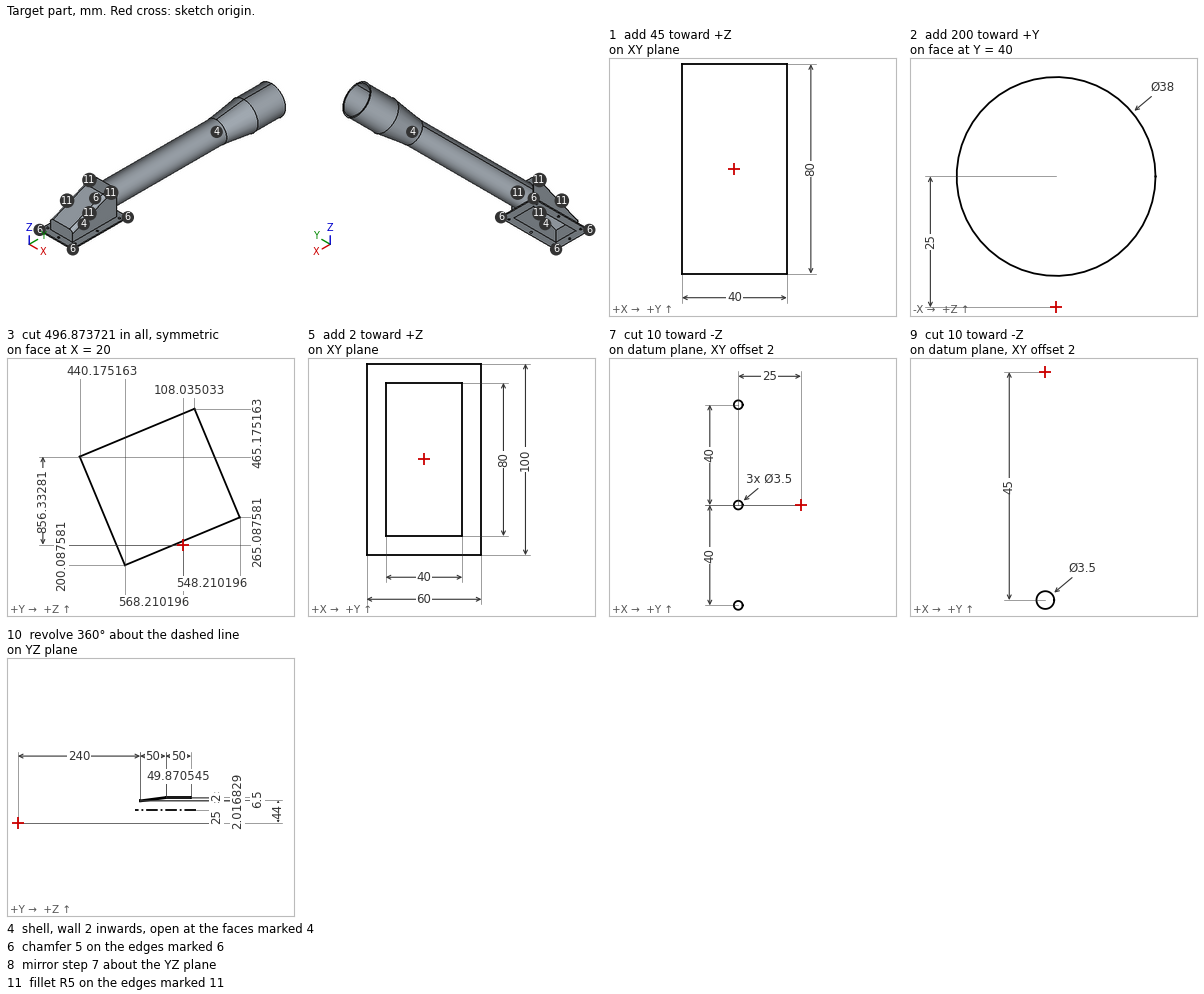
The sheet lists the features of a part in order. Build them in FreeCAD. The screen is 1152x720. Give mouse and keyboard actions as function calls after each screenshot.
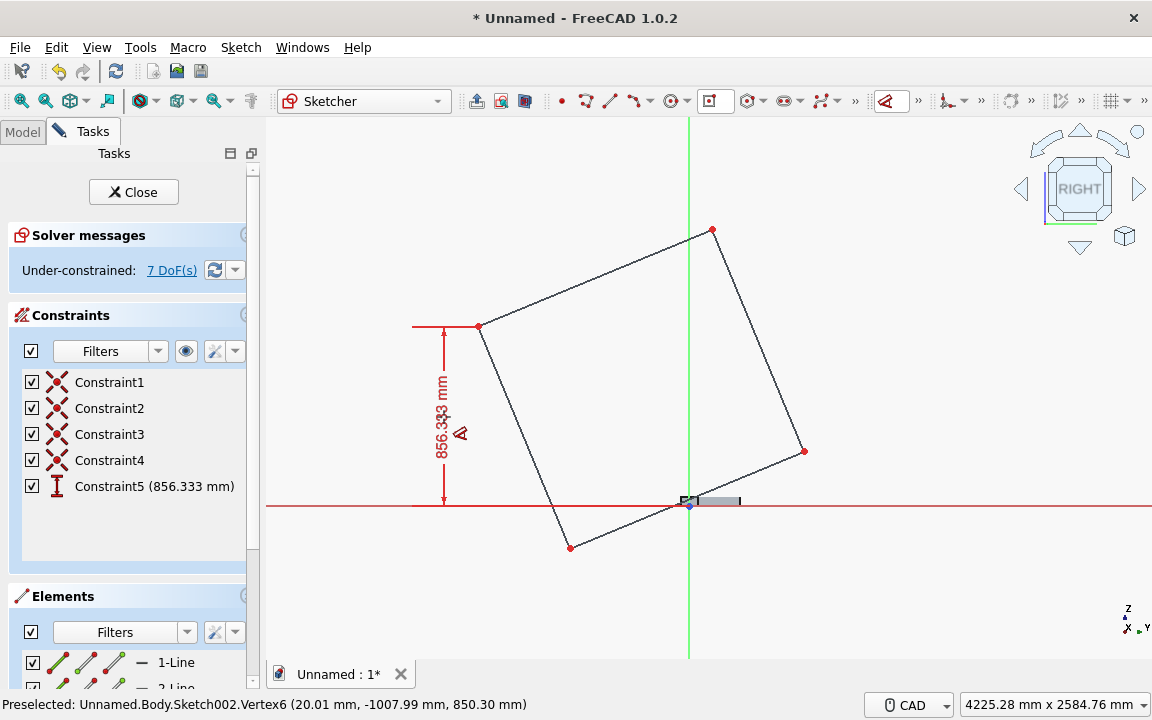
click(570, 549)
click(630, 583)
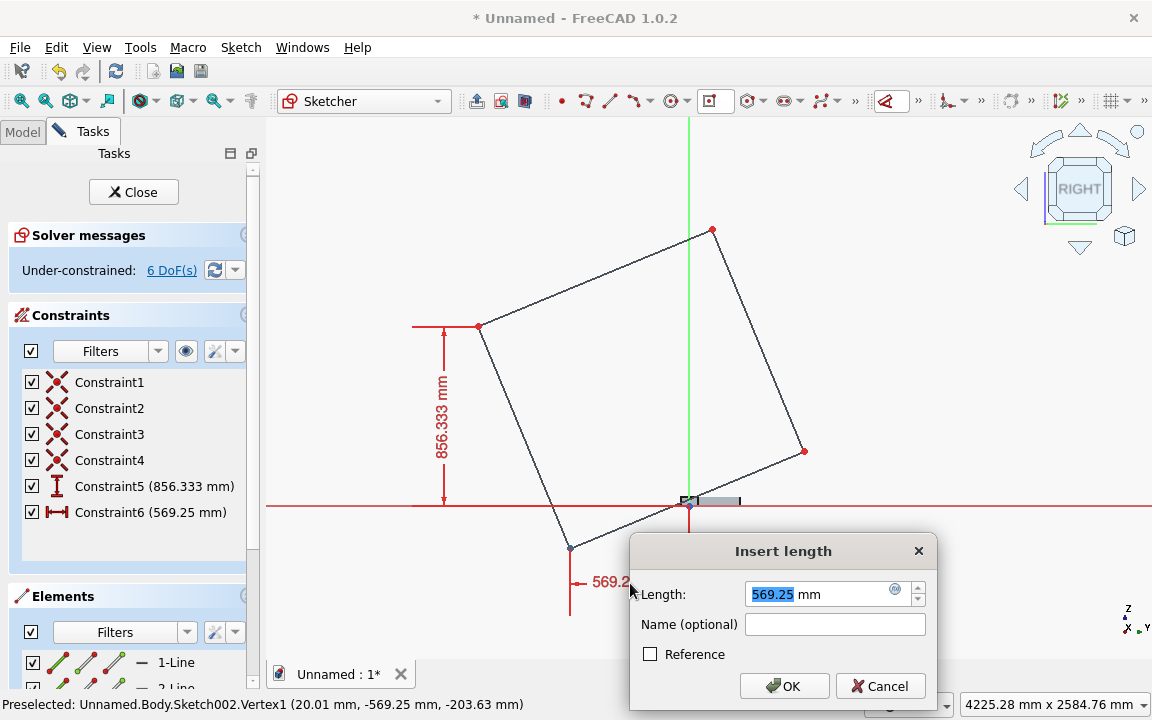
text(568.210196)
key(Return)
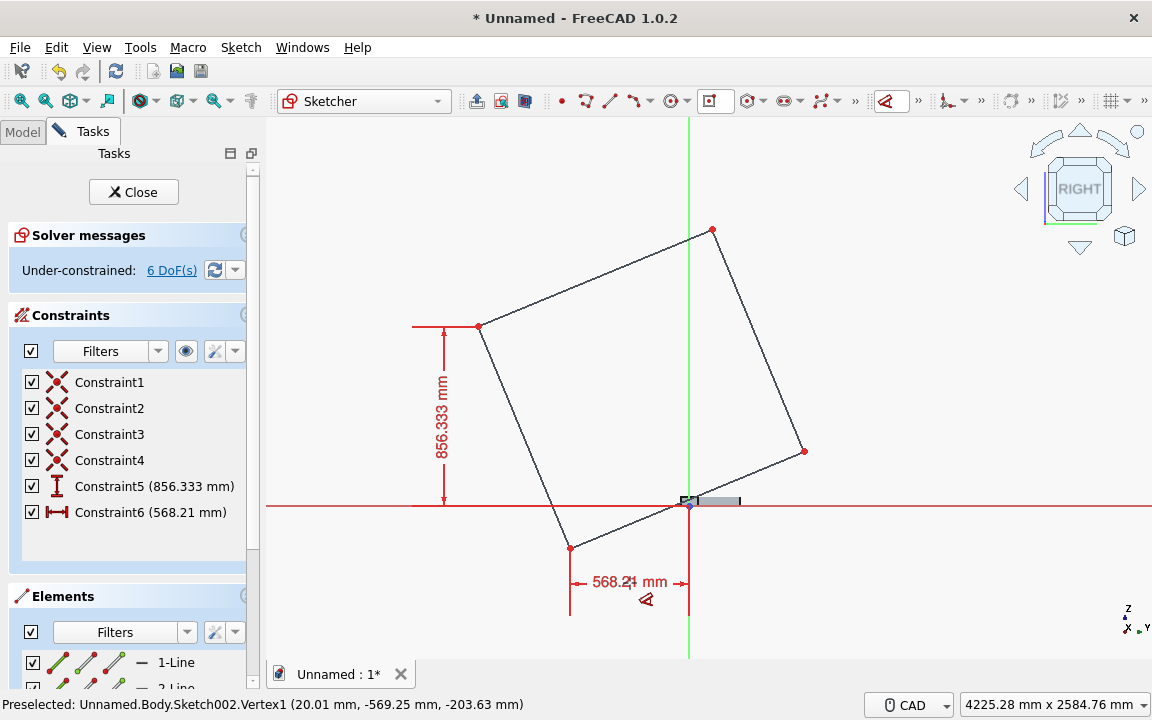
click(570, 549)
click(536, 528)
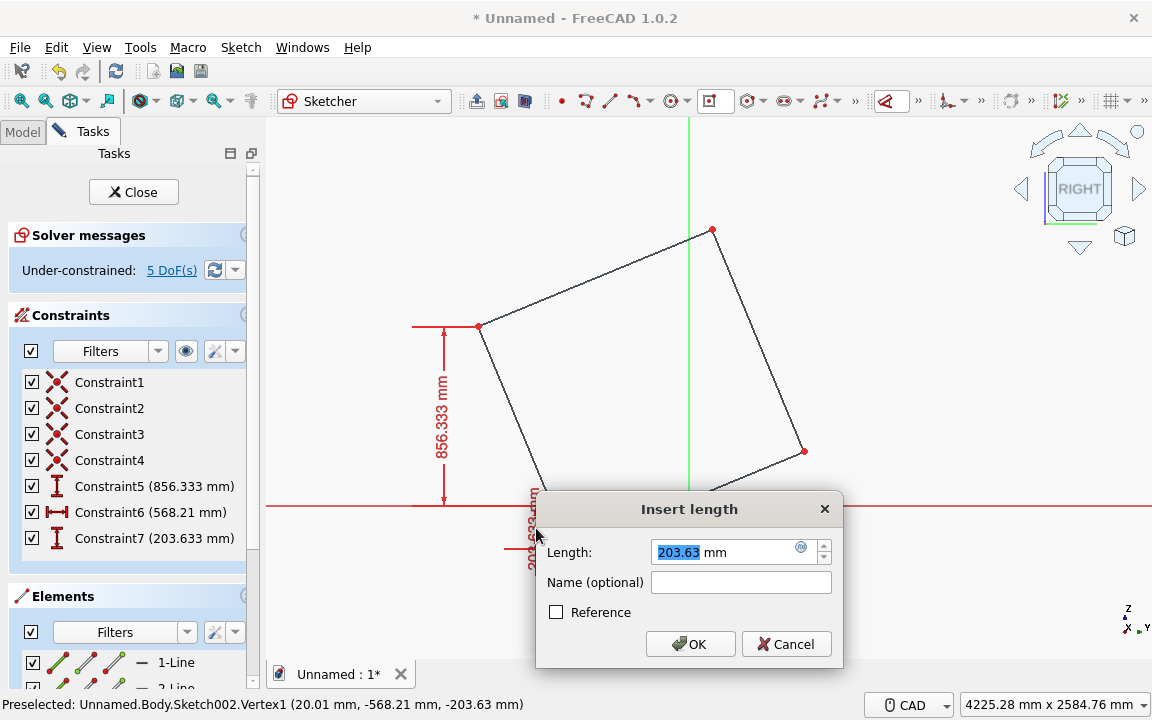
text(200.087581)
key(Return)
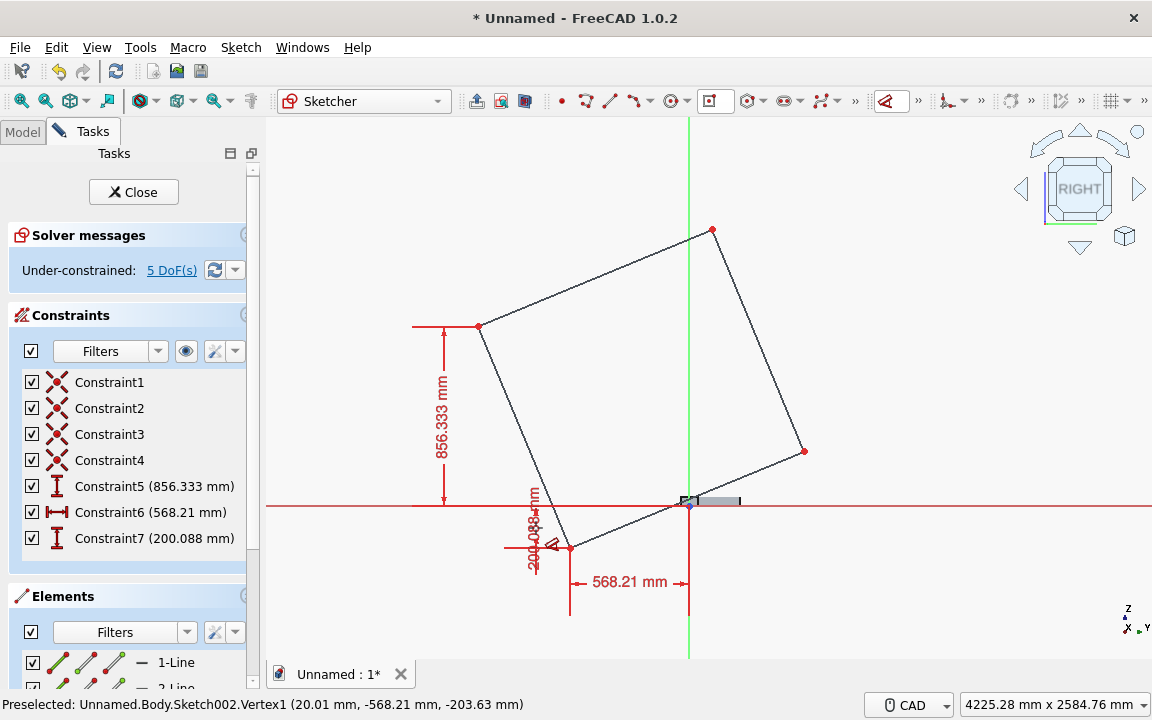
click(804, 452)
click(747, 540)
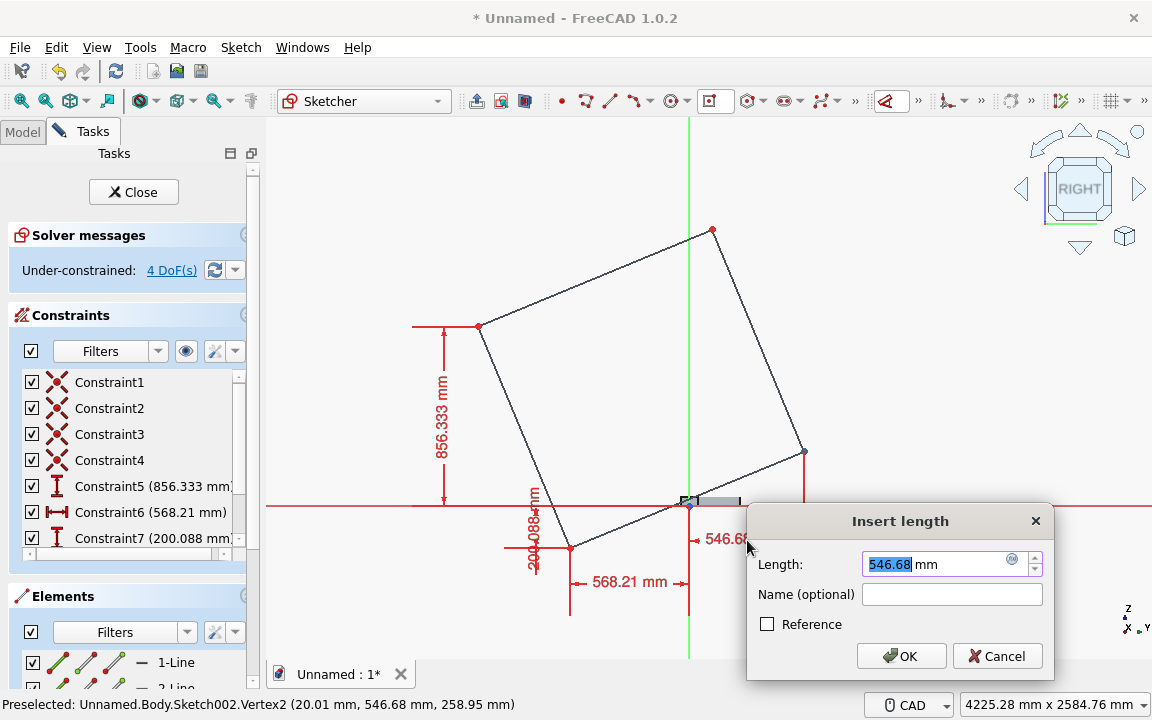
text(548.210196)
key(Return)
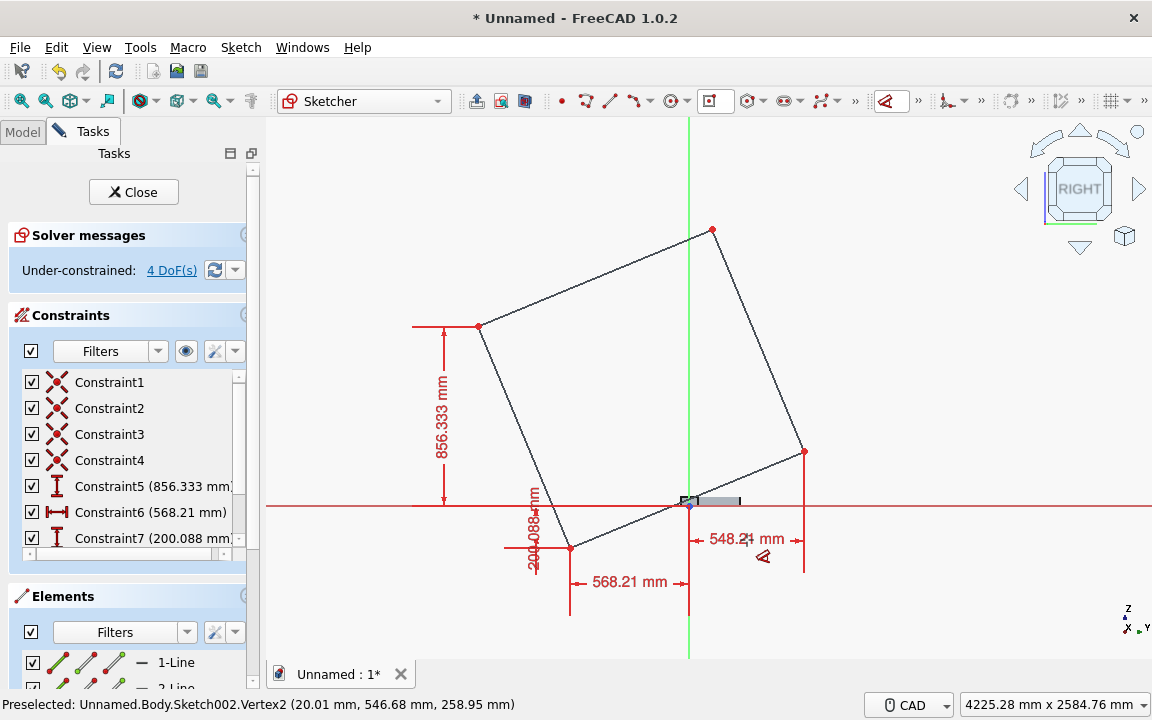
click(804, 452)
click(838, 479)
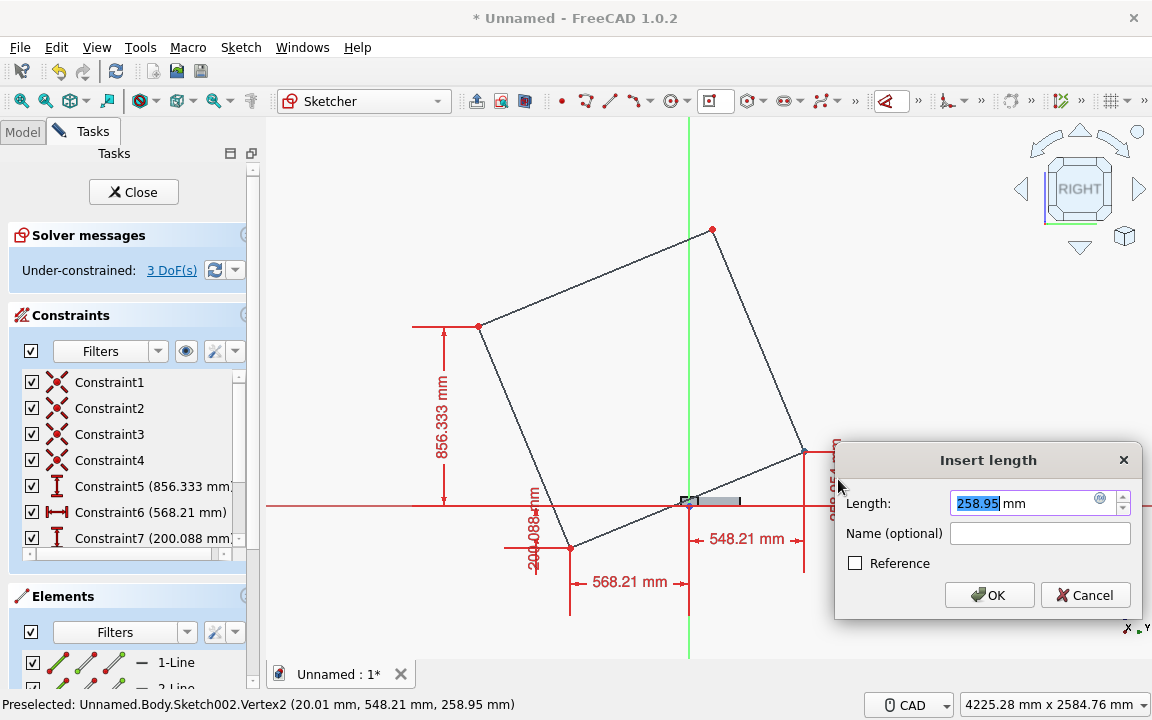
text(265.087581)
key(Return)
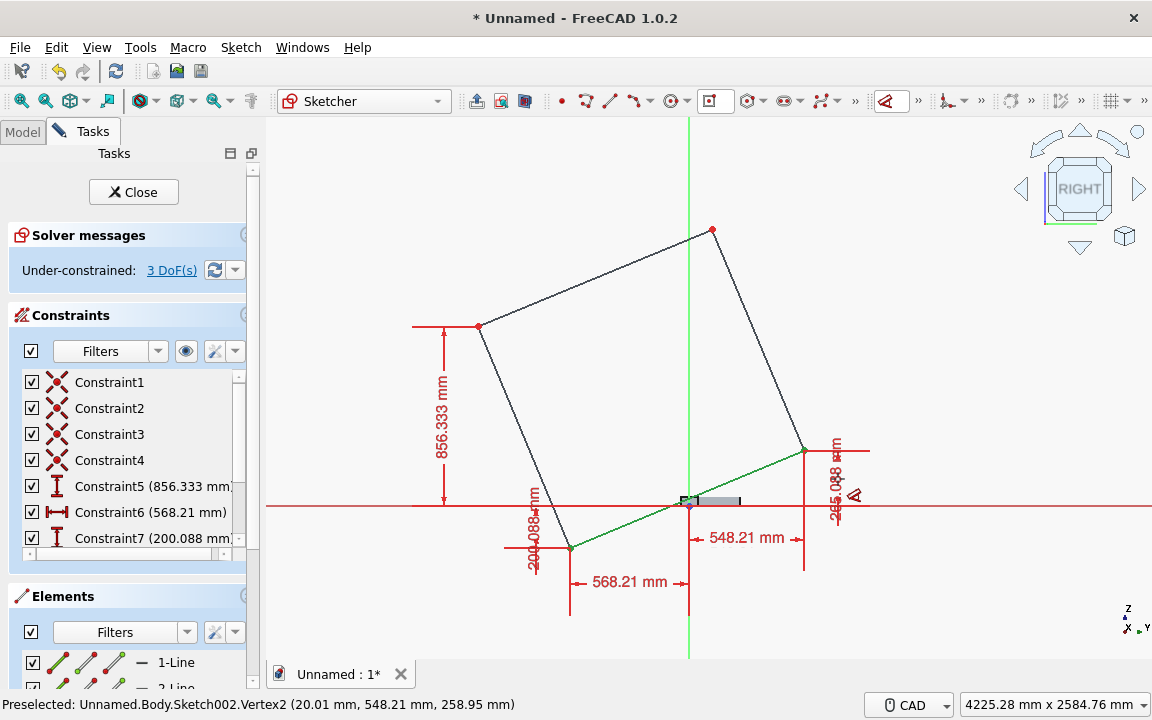
scroll(712, 230, up, 3)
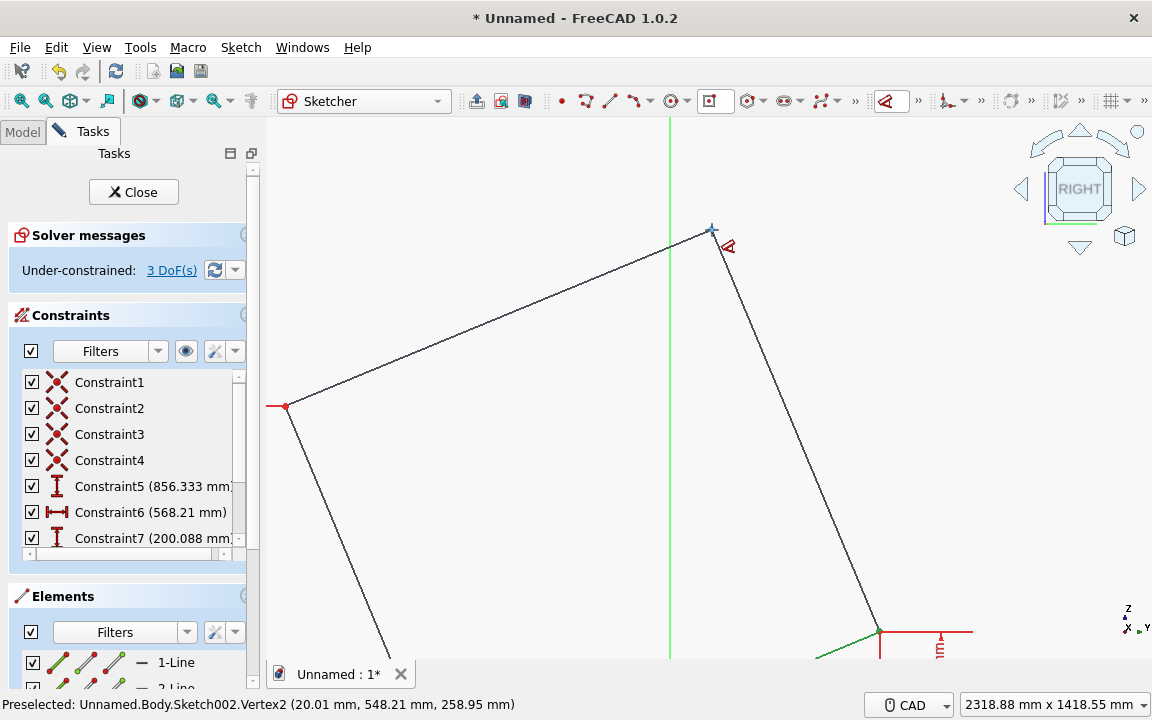
click(712, 230)
click(691, 196)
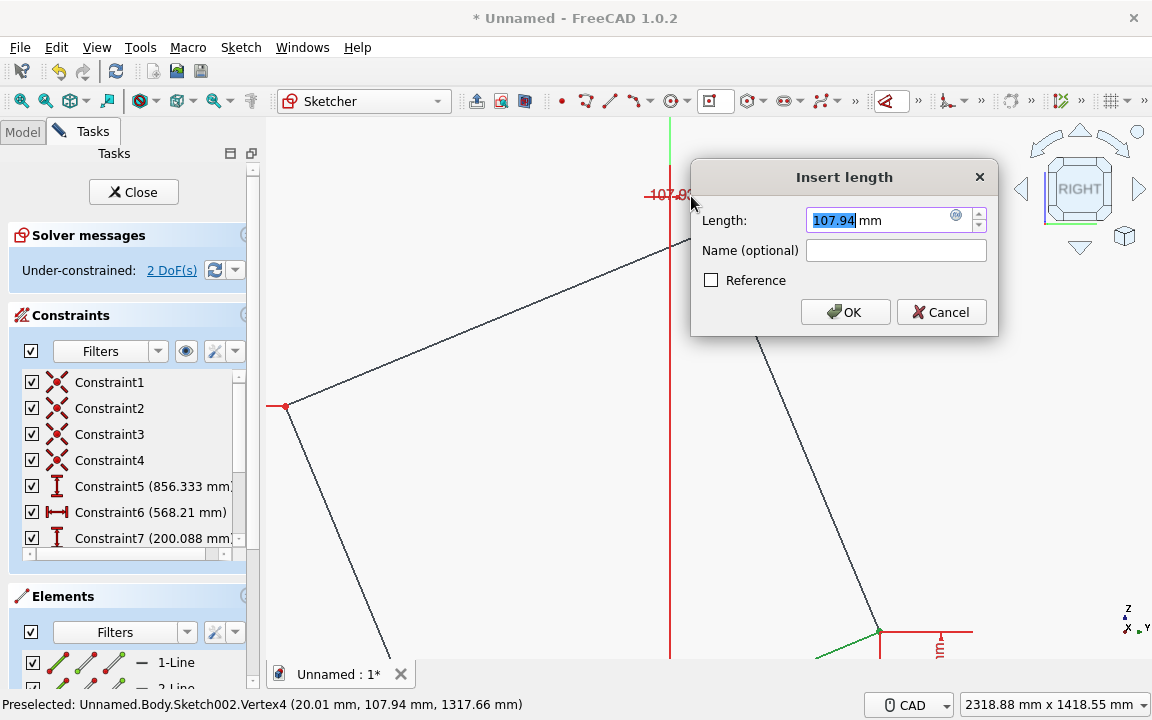
text(108.035033)
key(Return)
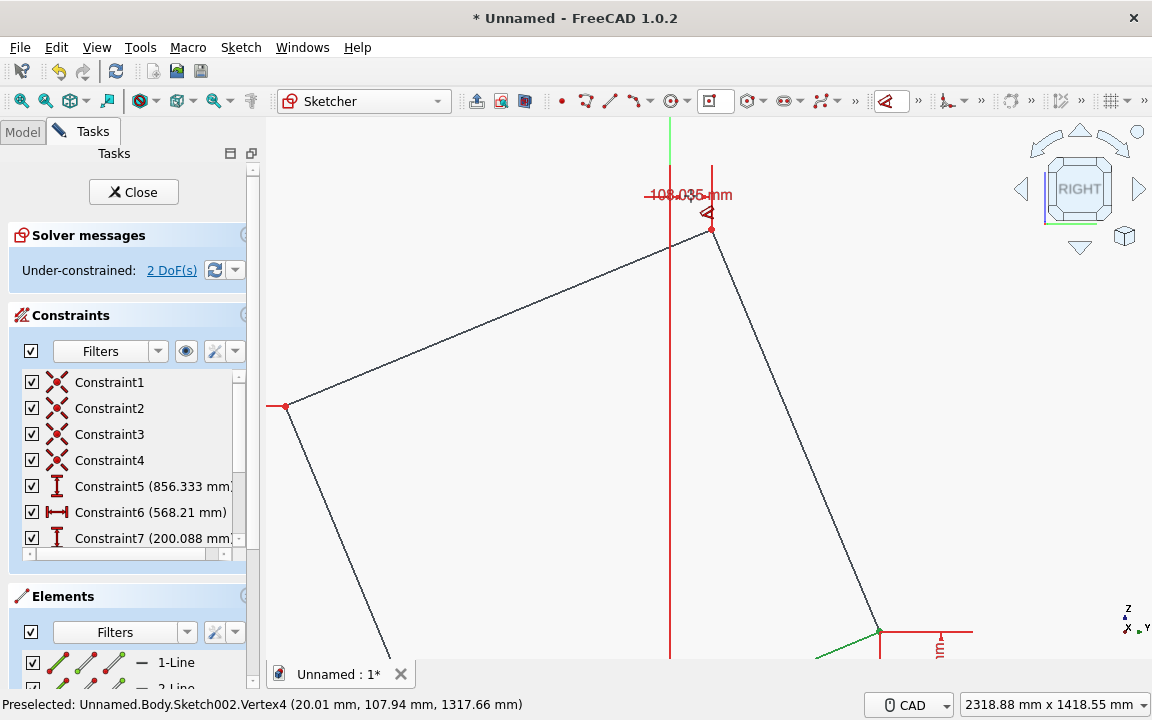
click(584, 283)
click(746, 277)